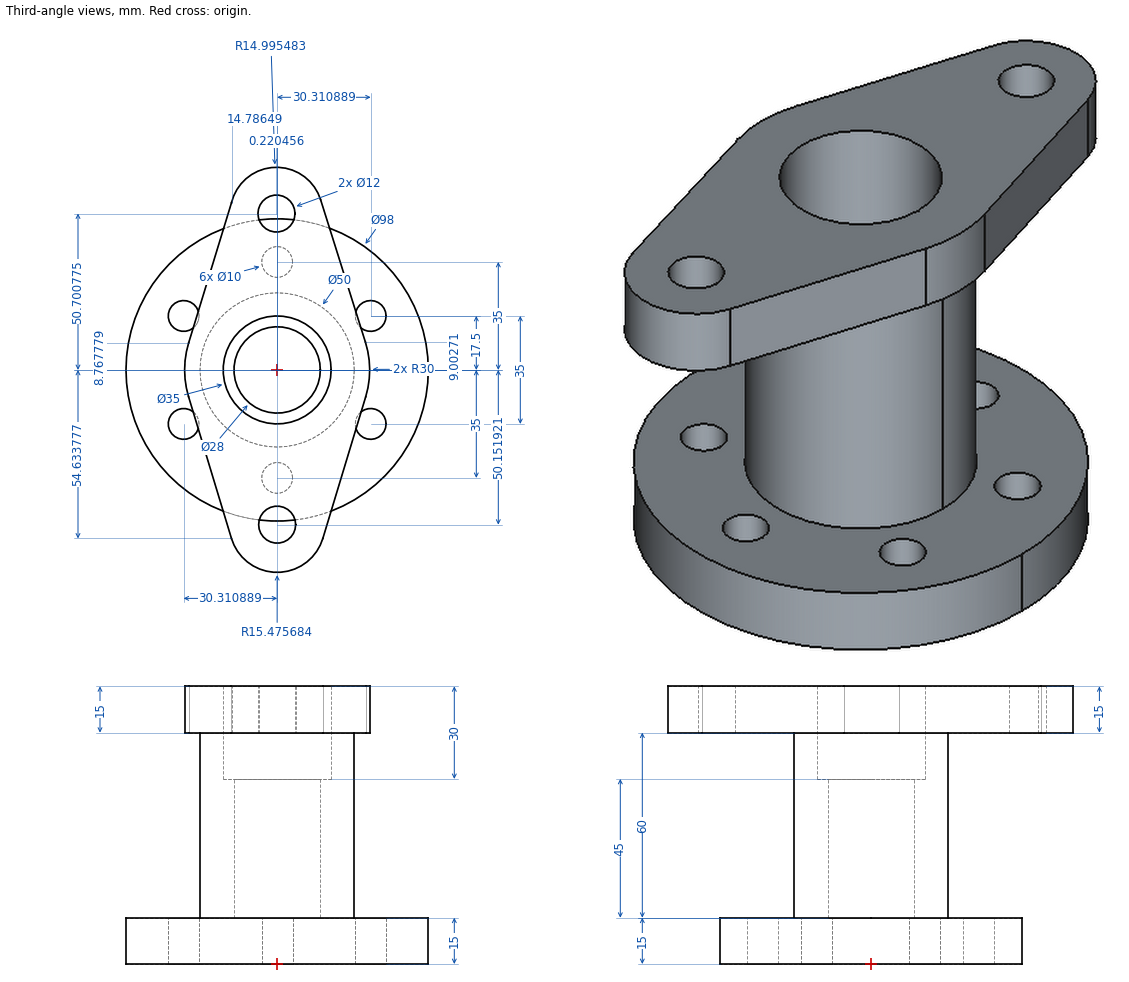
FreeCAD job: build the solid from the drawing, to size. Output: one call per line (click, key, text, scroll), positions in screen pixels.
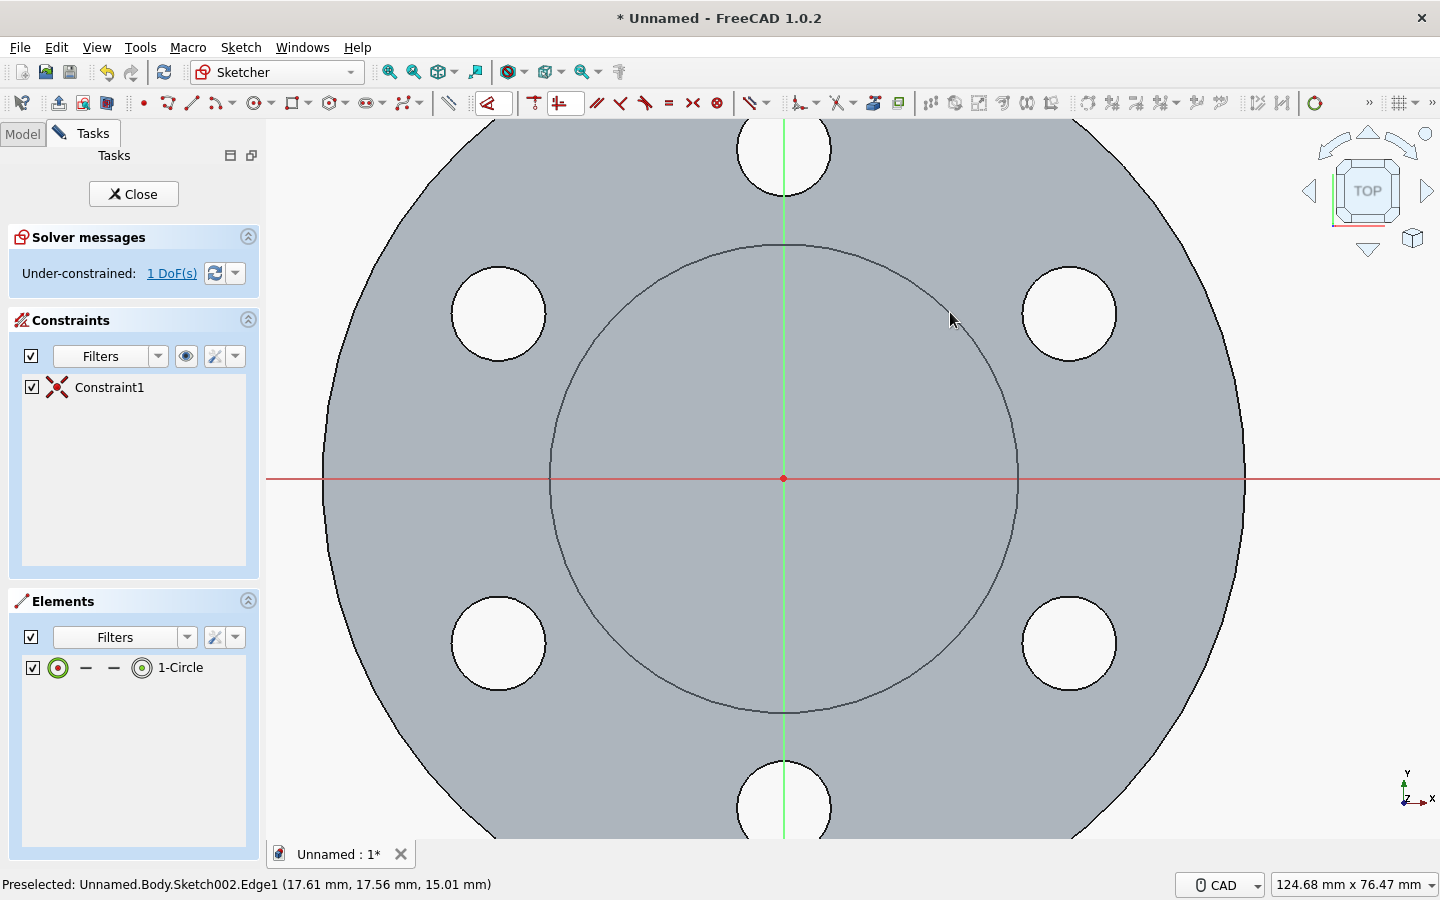
click(949, 312)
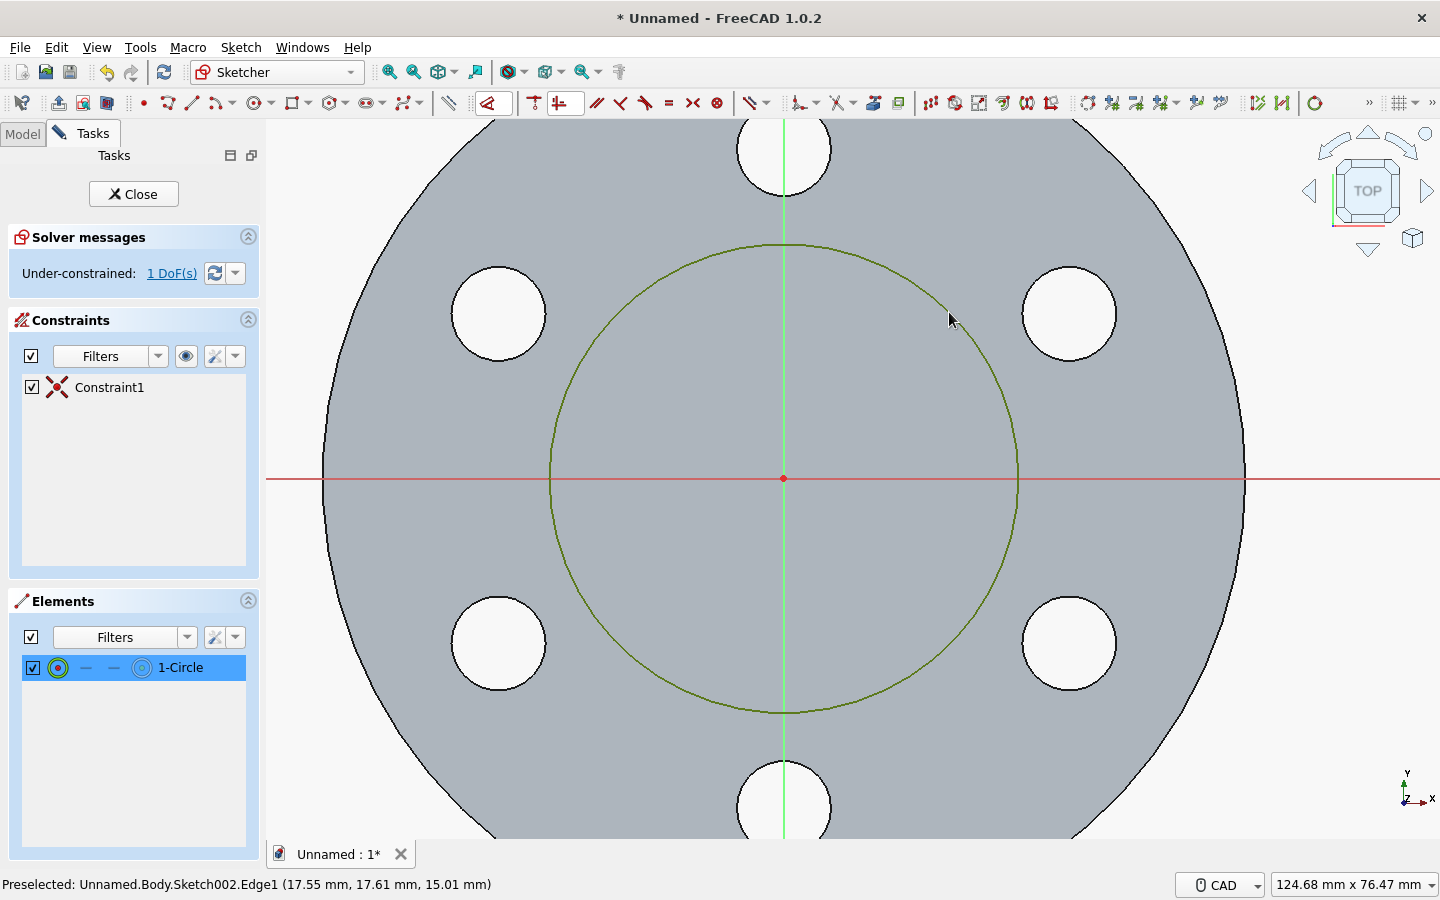
key(k)
key(o)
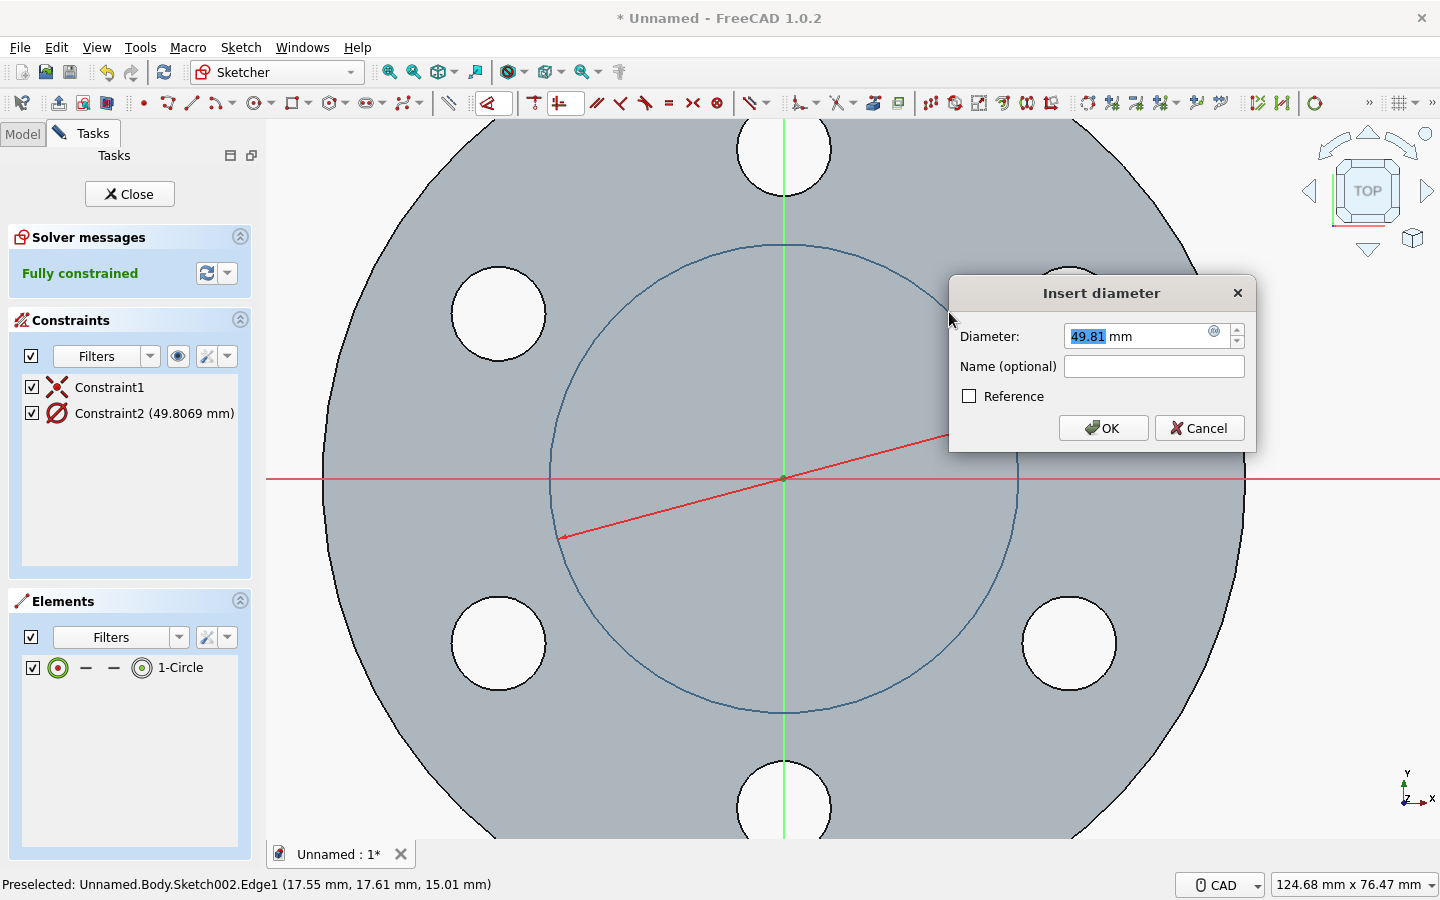
text(50)
key(Return)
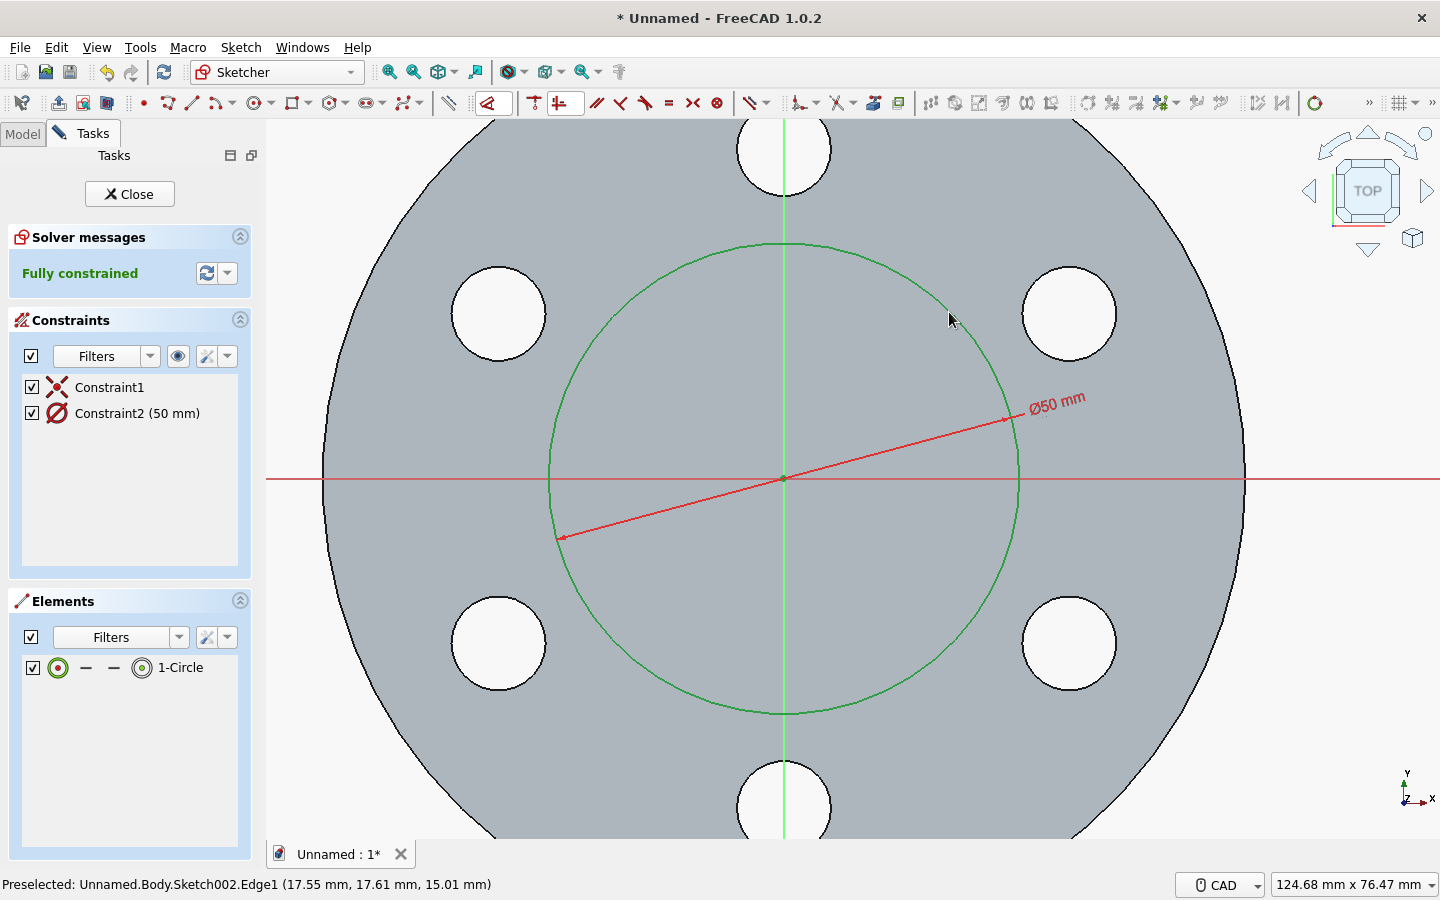
click(130, 194)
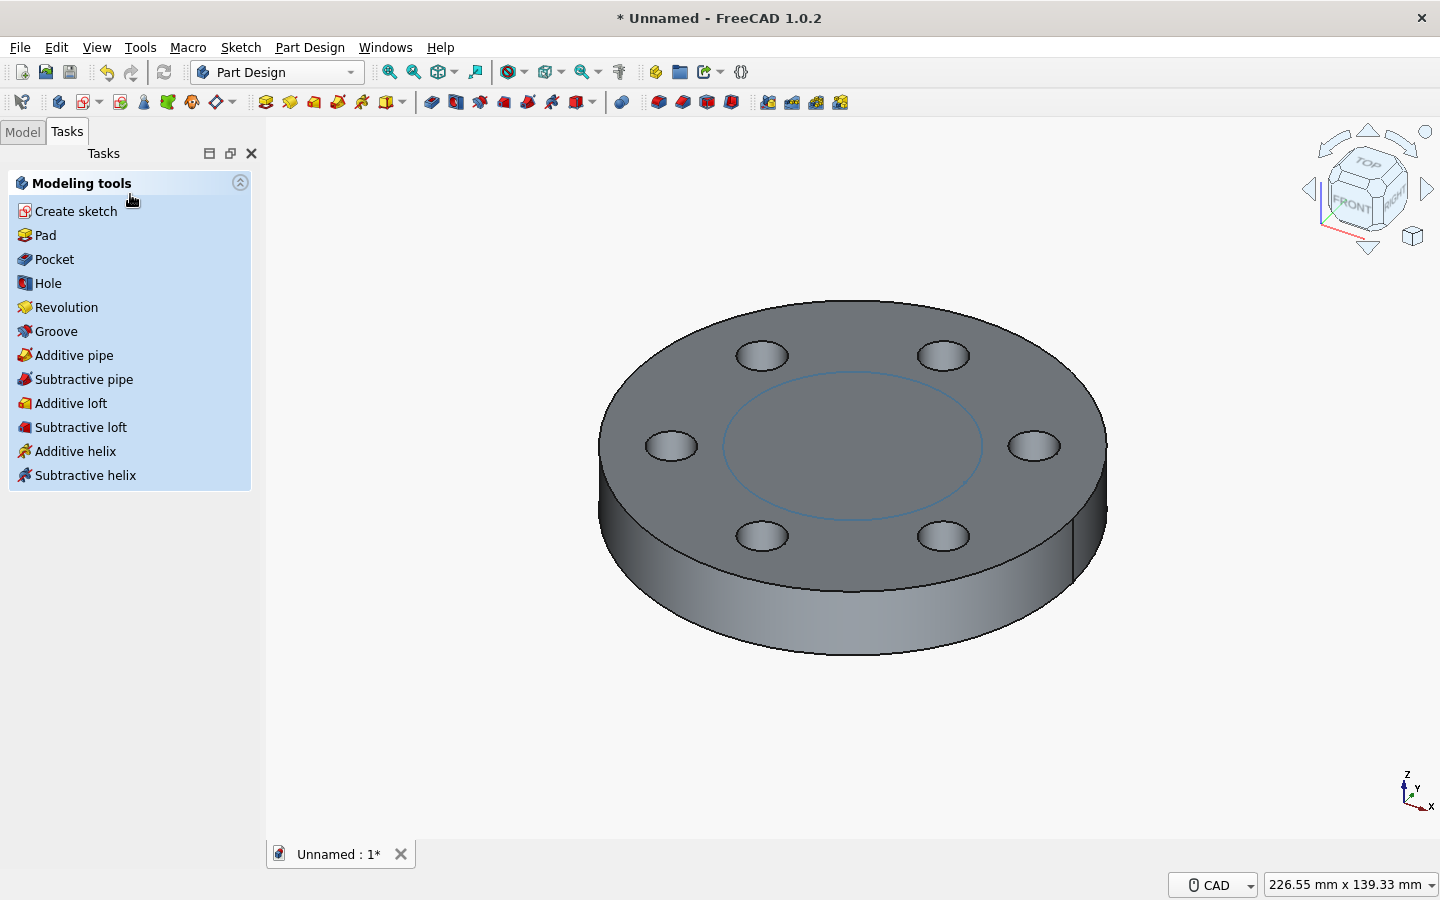
click(266, 102)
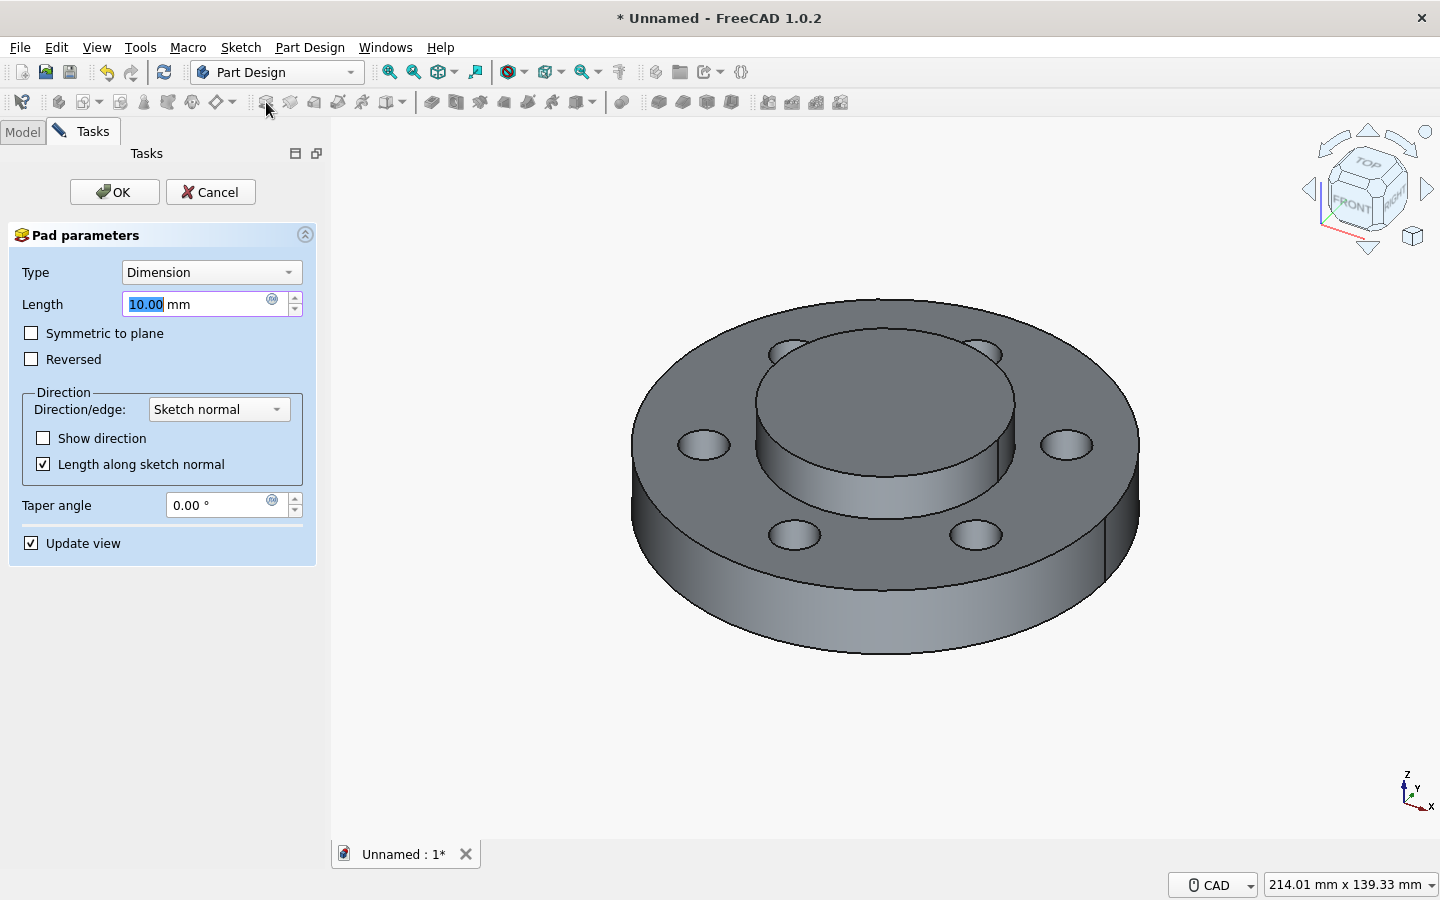
text(60)
key(Tab)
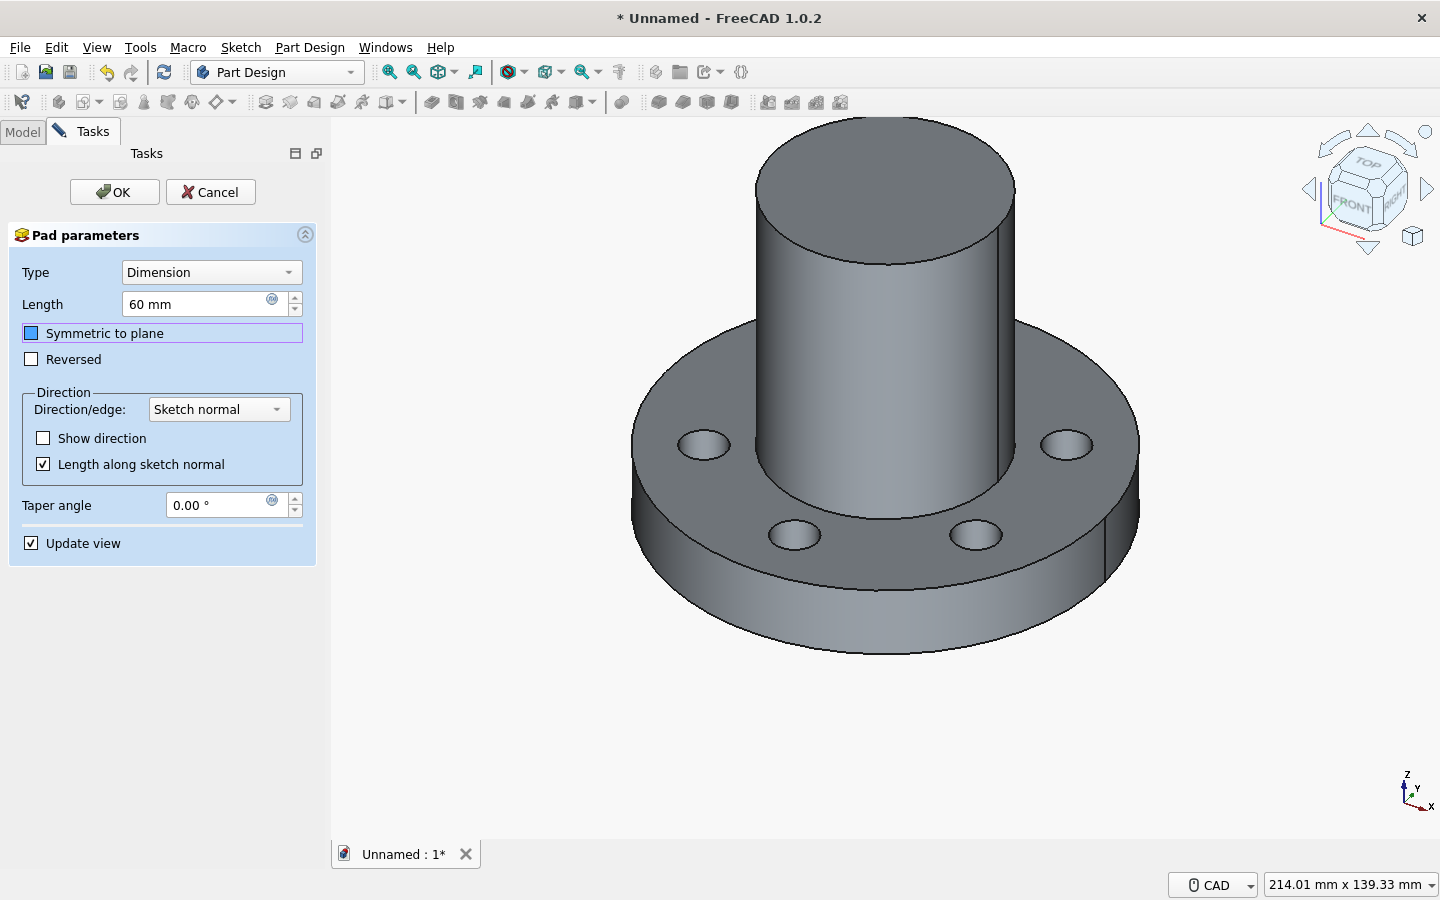
click(115, 192)